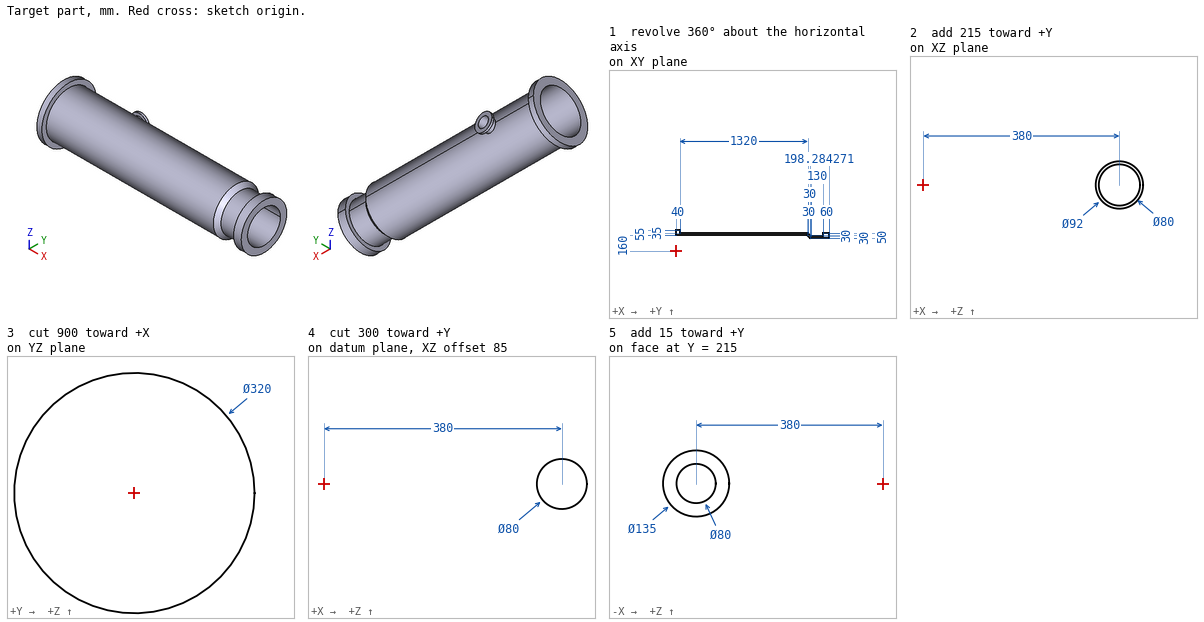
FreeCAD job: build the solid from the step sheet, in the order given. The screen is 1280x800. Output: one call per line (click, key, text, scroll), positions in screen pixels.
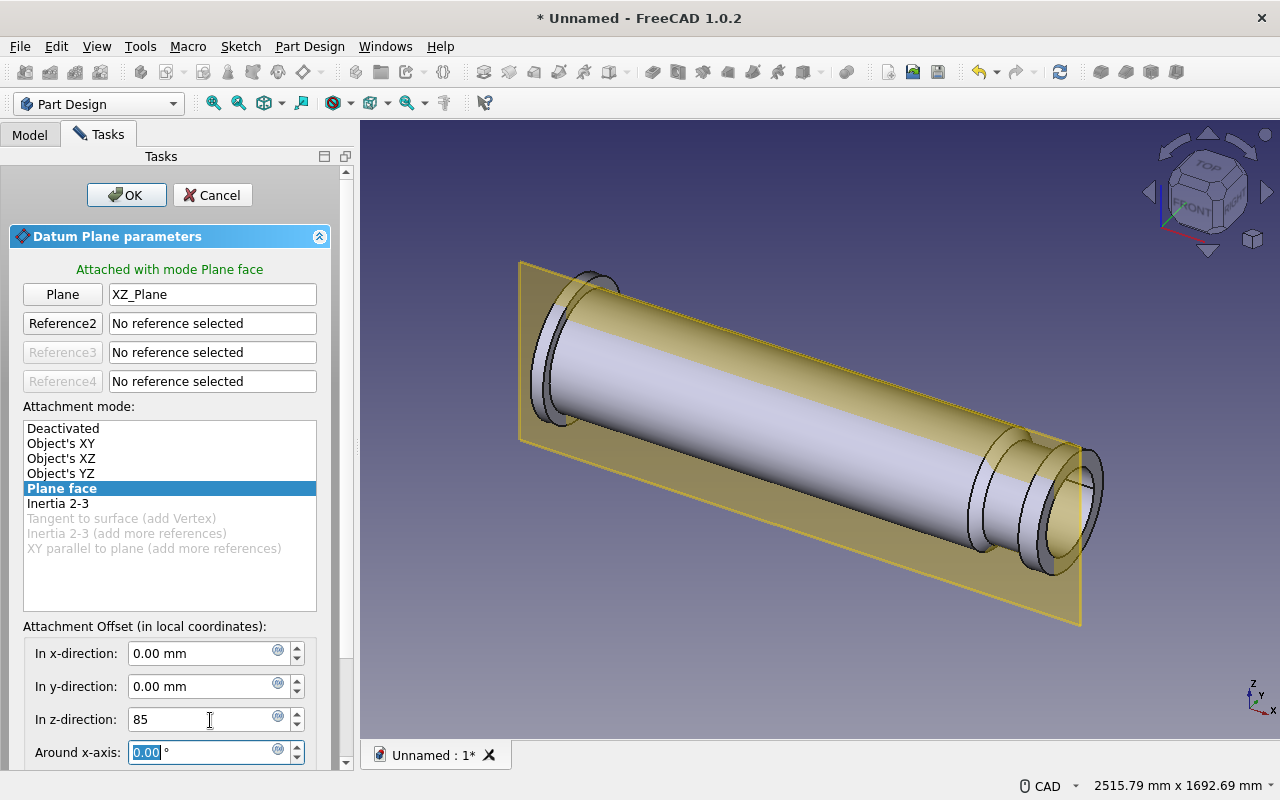
click(127, 195)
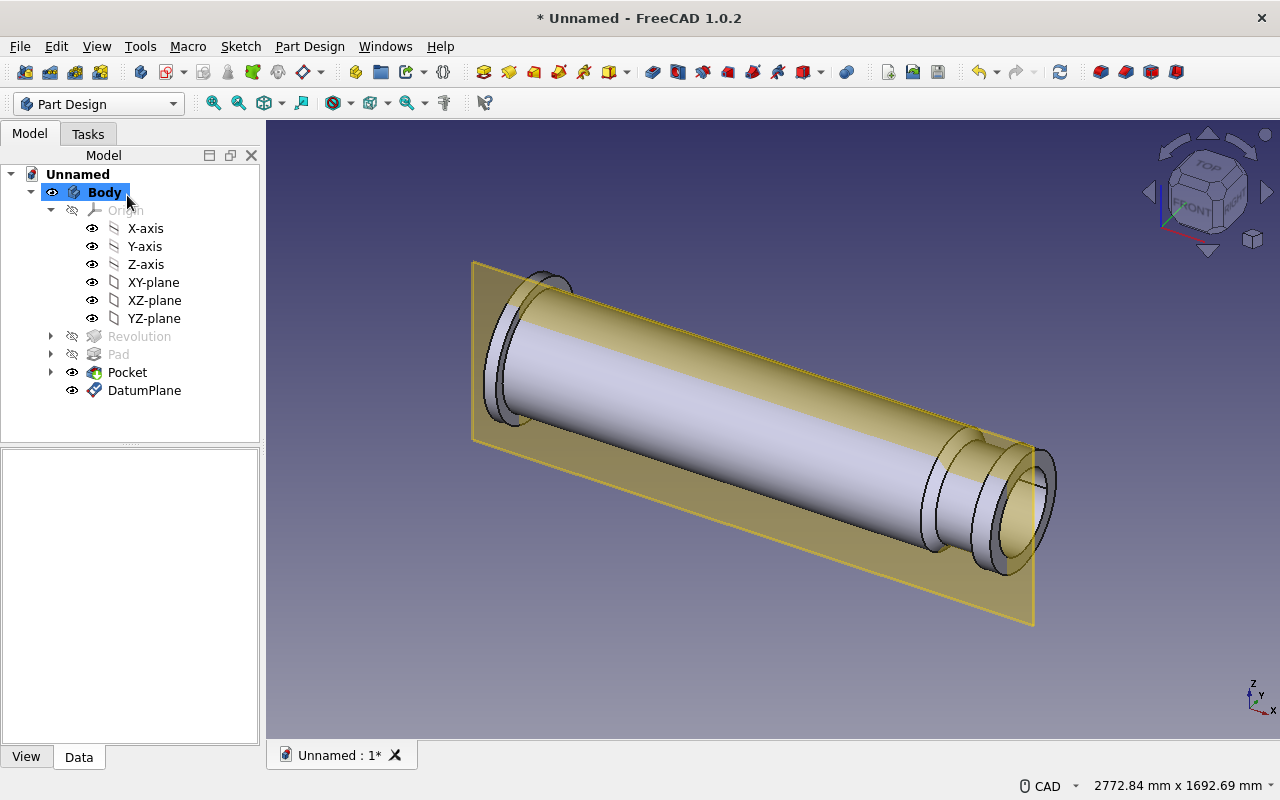
click(117, 390)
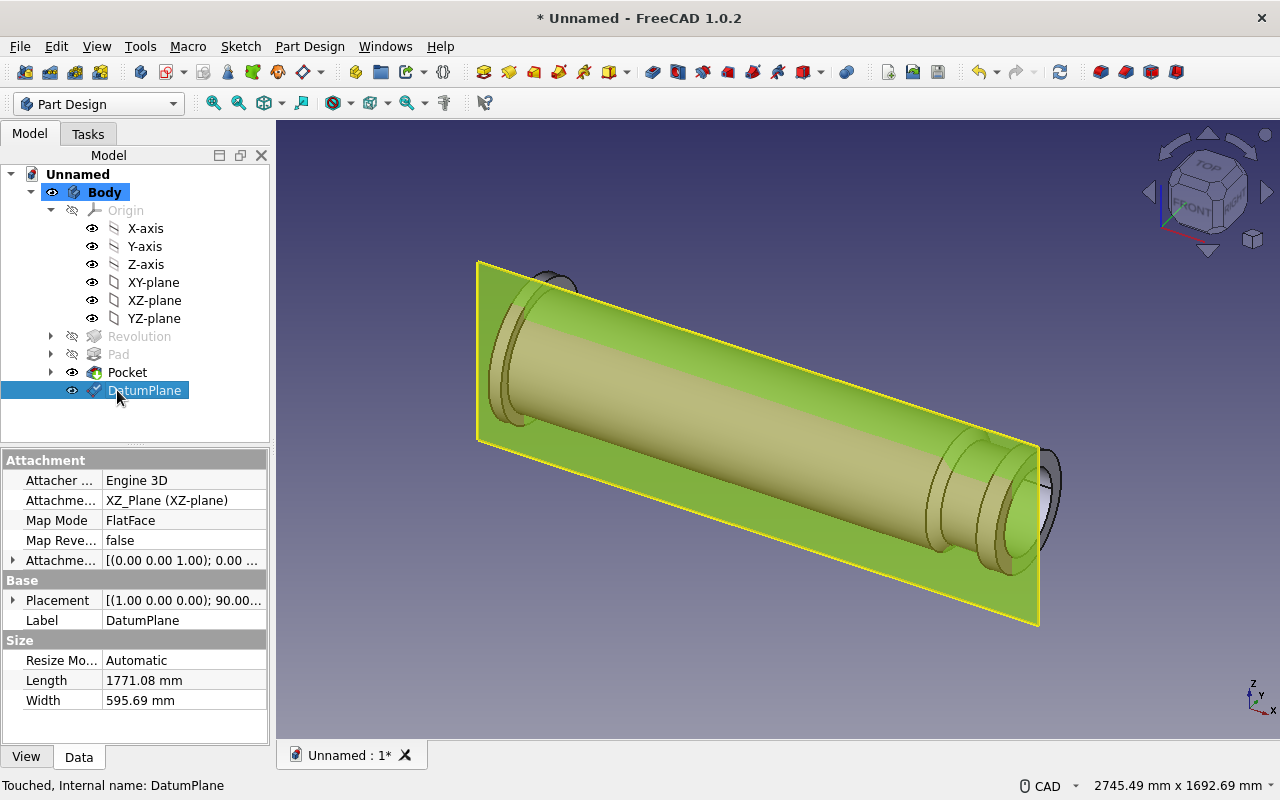
click(166, 72)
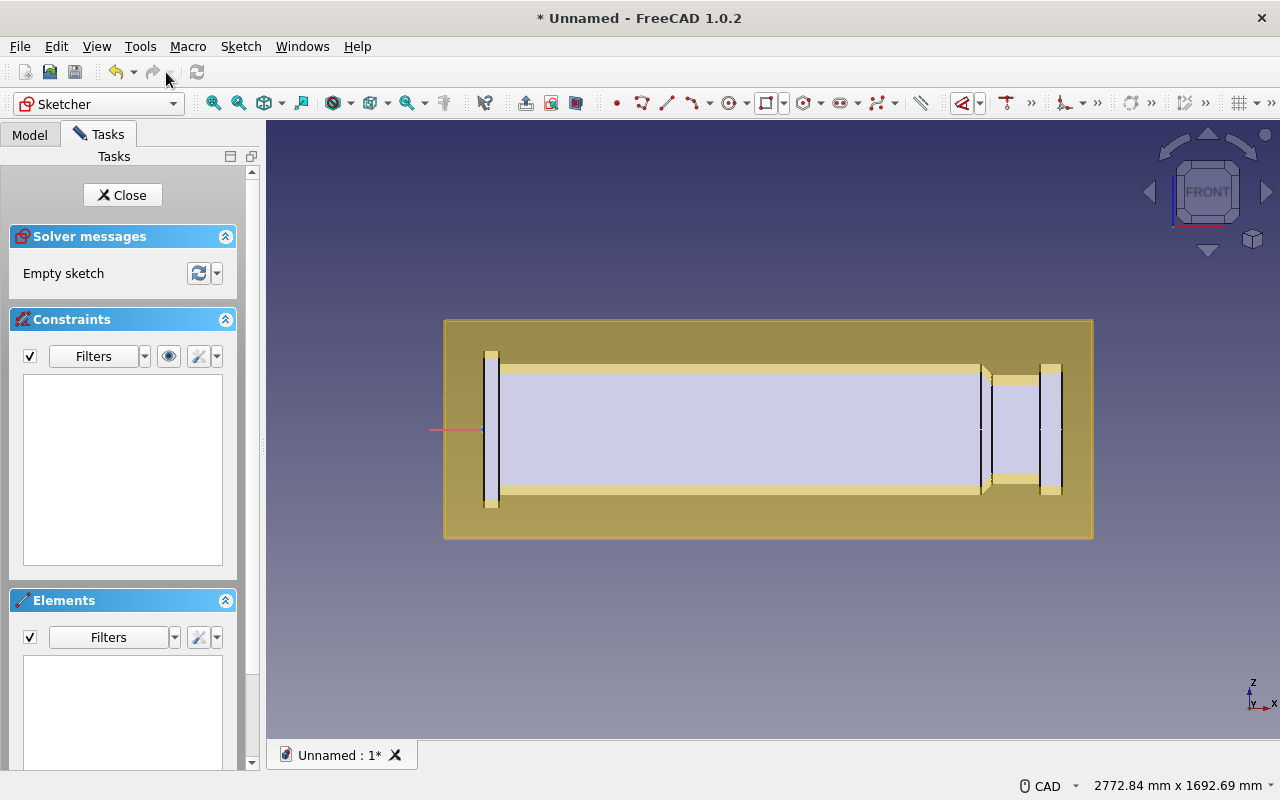
key(q)
key(s)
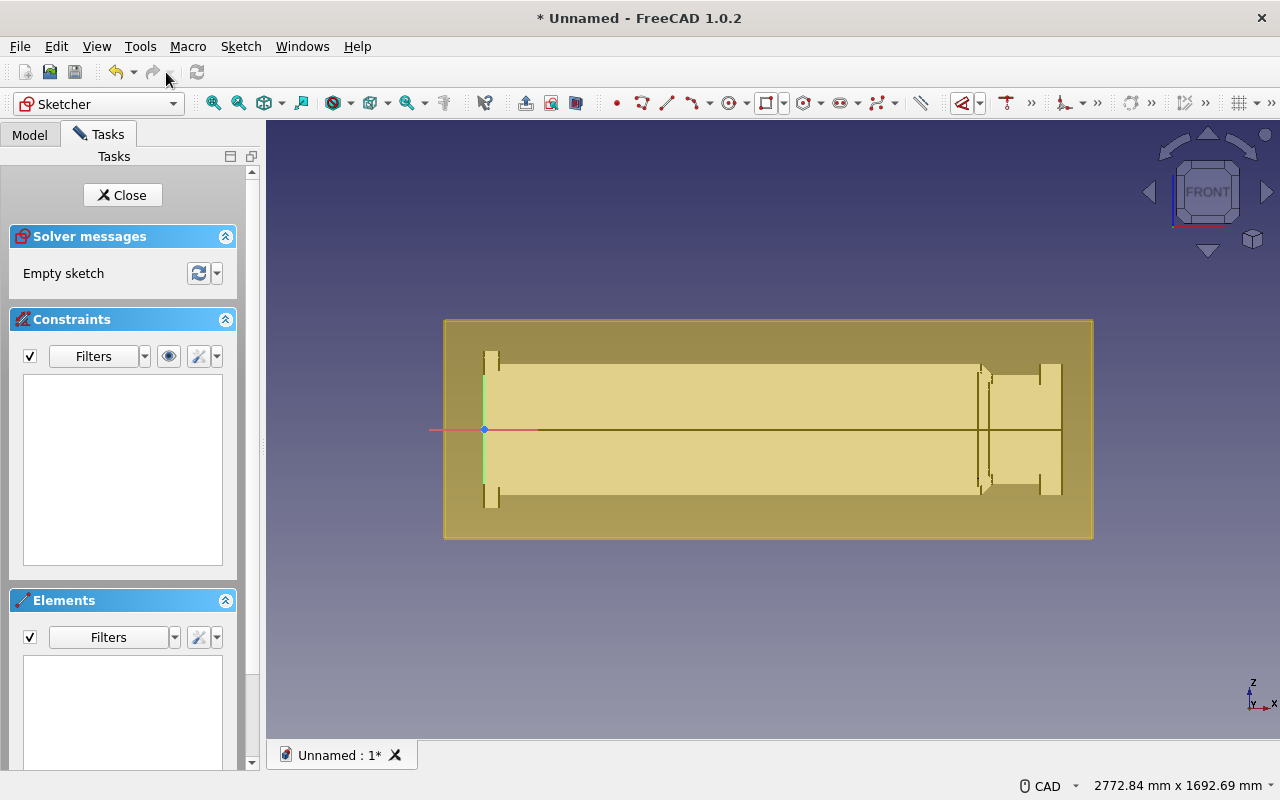
scroll(617, 430, up, 13)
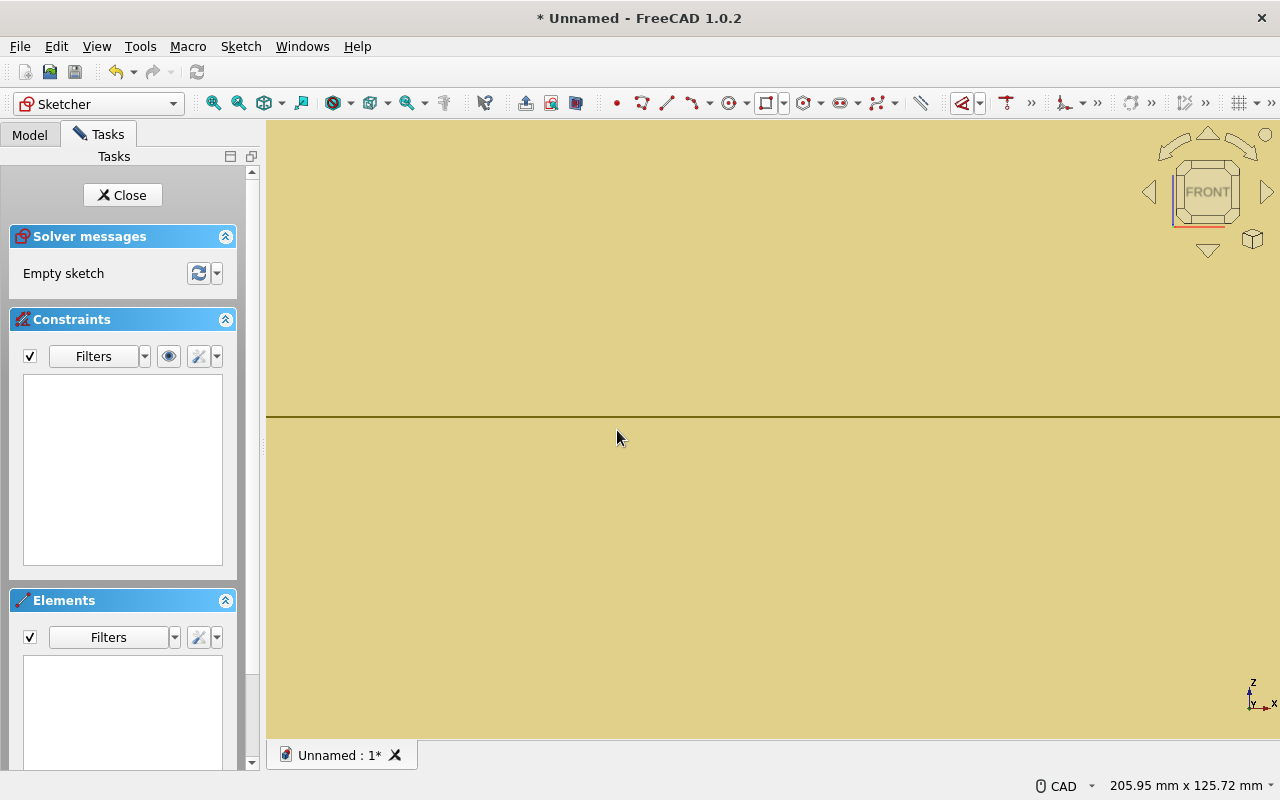
click(728, 104)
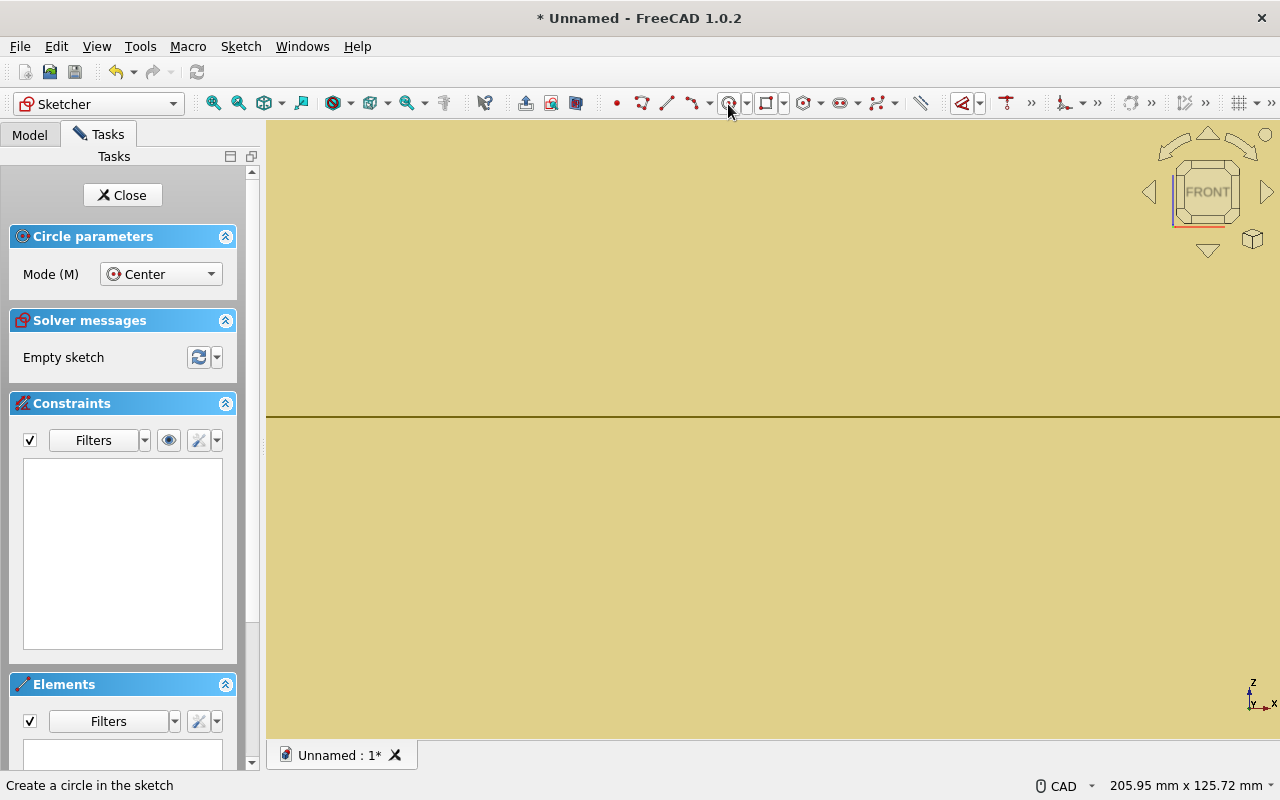
click(694, 417)
move(834, 278)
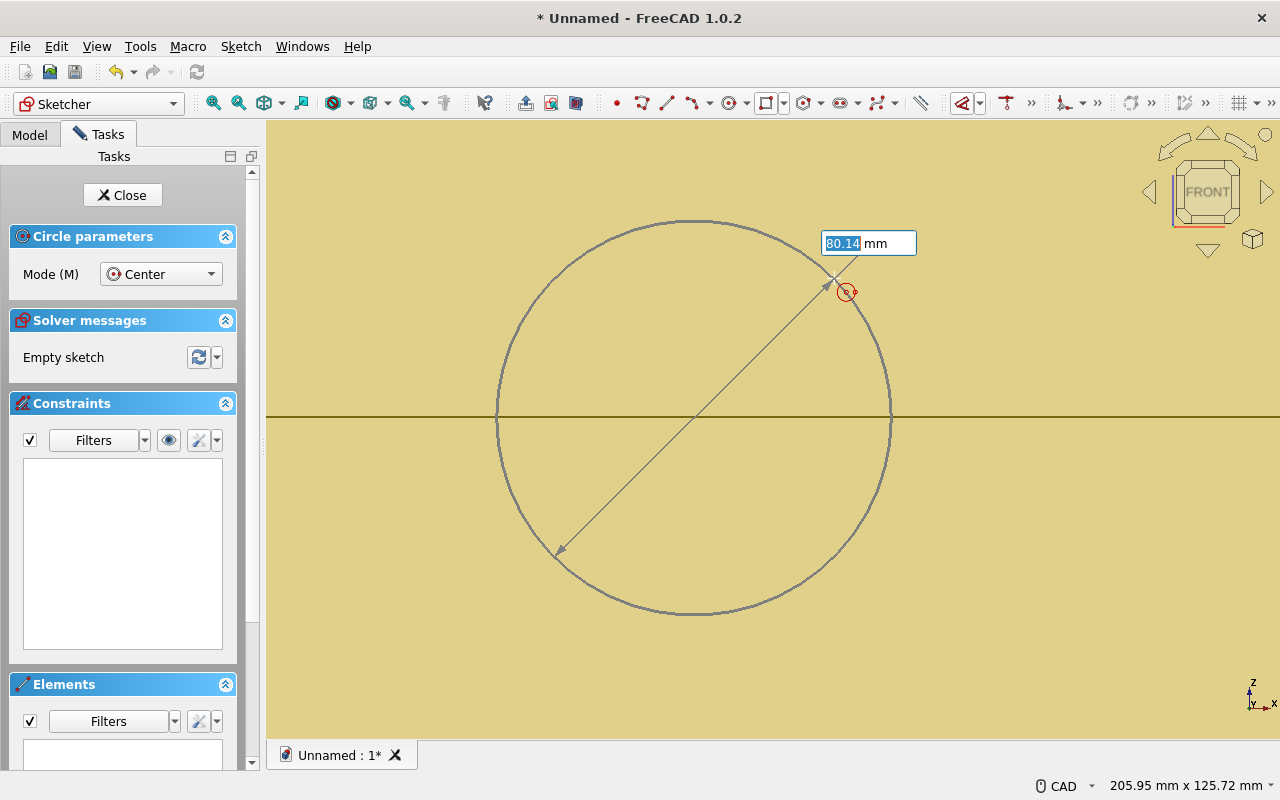
text(80)
key(Return)
key(Escape)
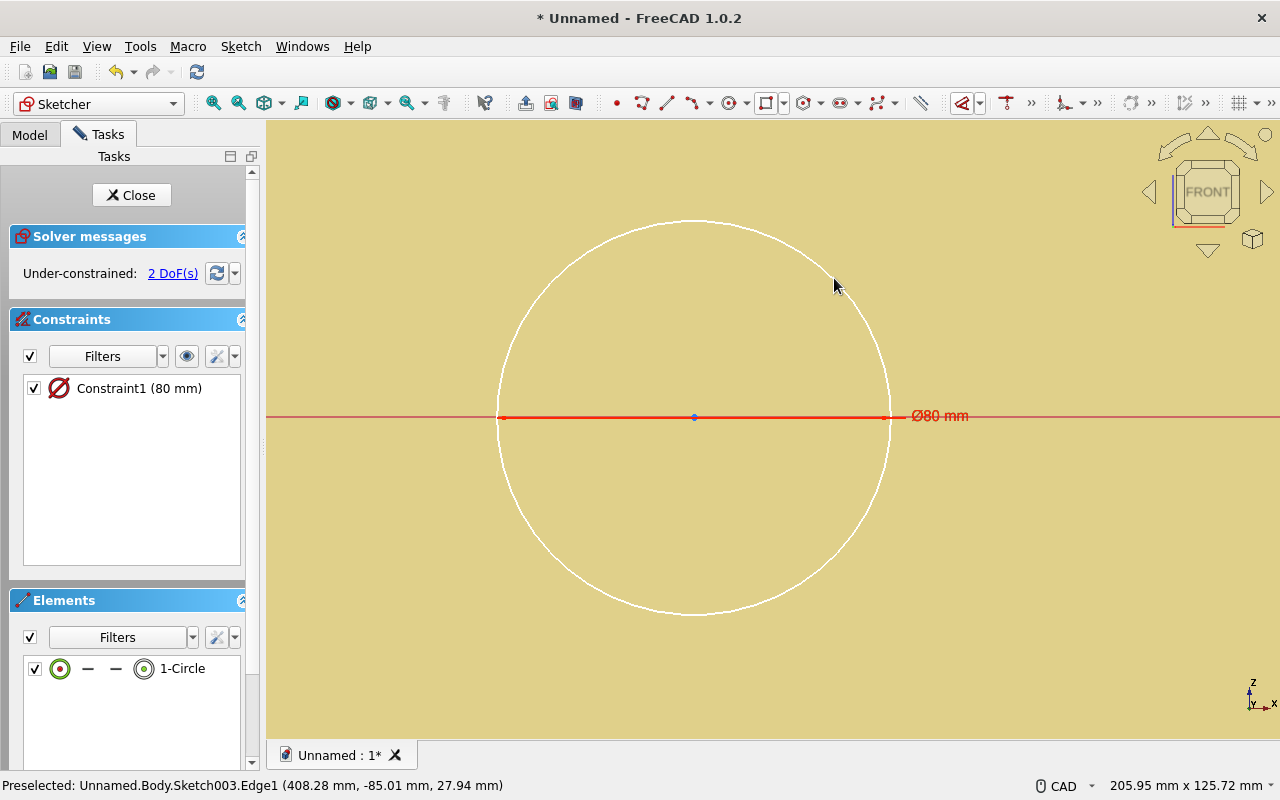
click(694, 418)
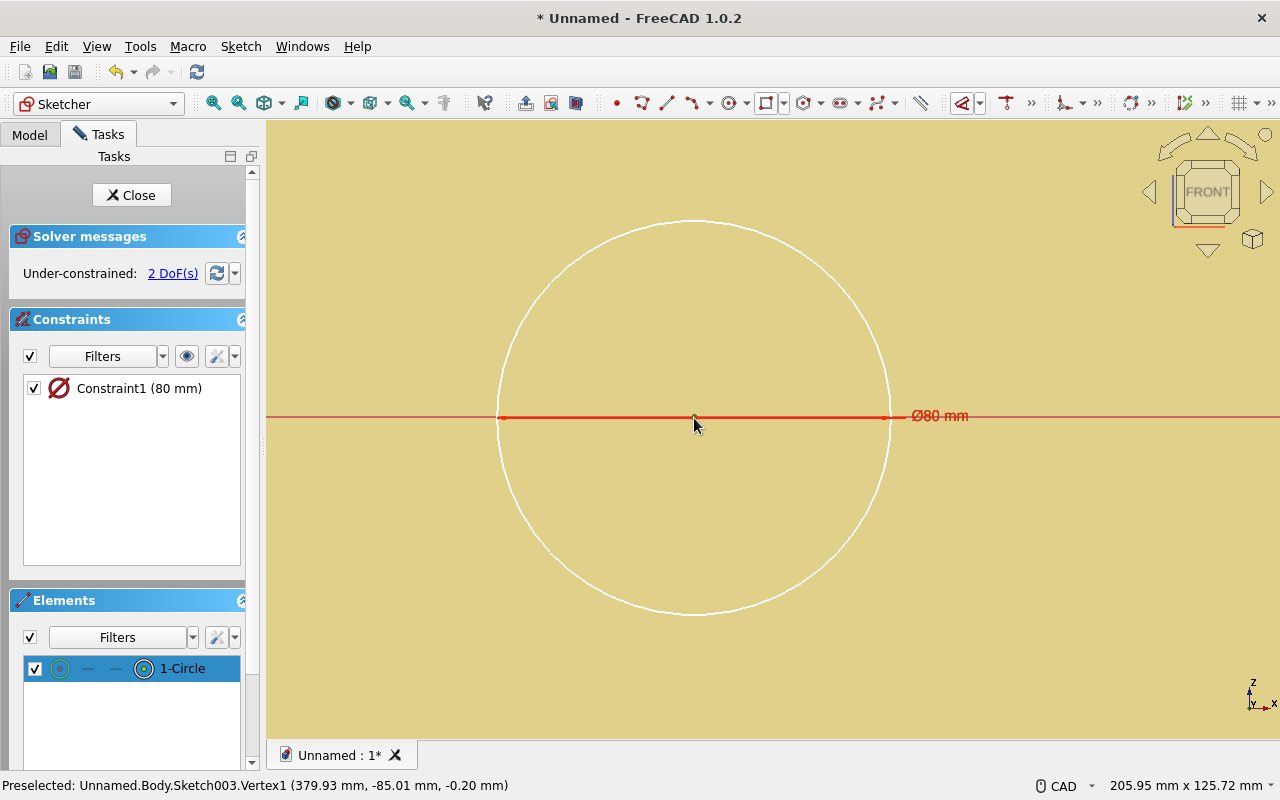
click(353, 417)